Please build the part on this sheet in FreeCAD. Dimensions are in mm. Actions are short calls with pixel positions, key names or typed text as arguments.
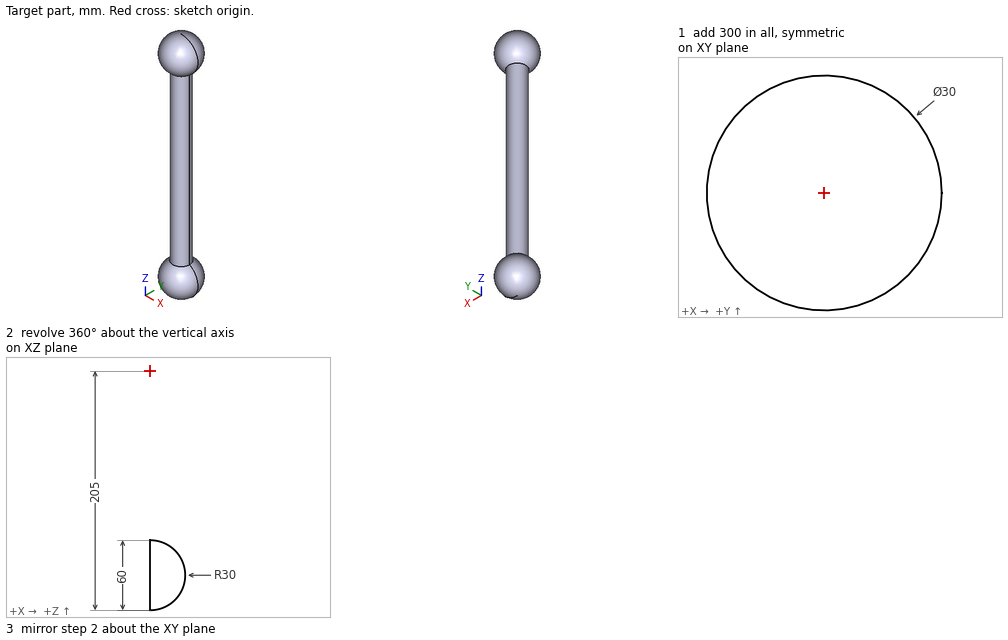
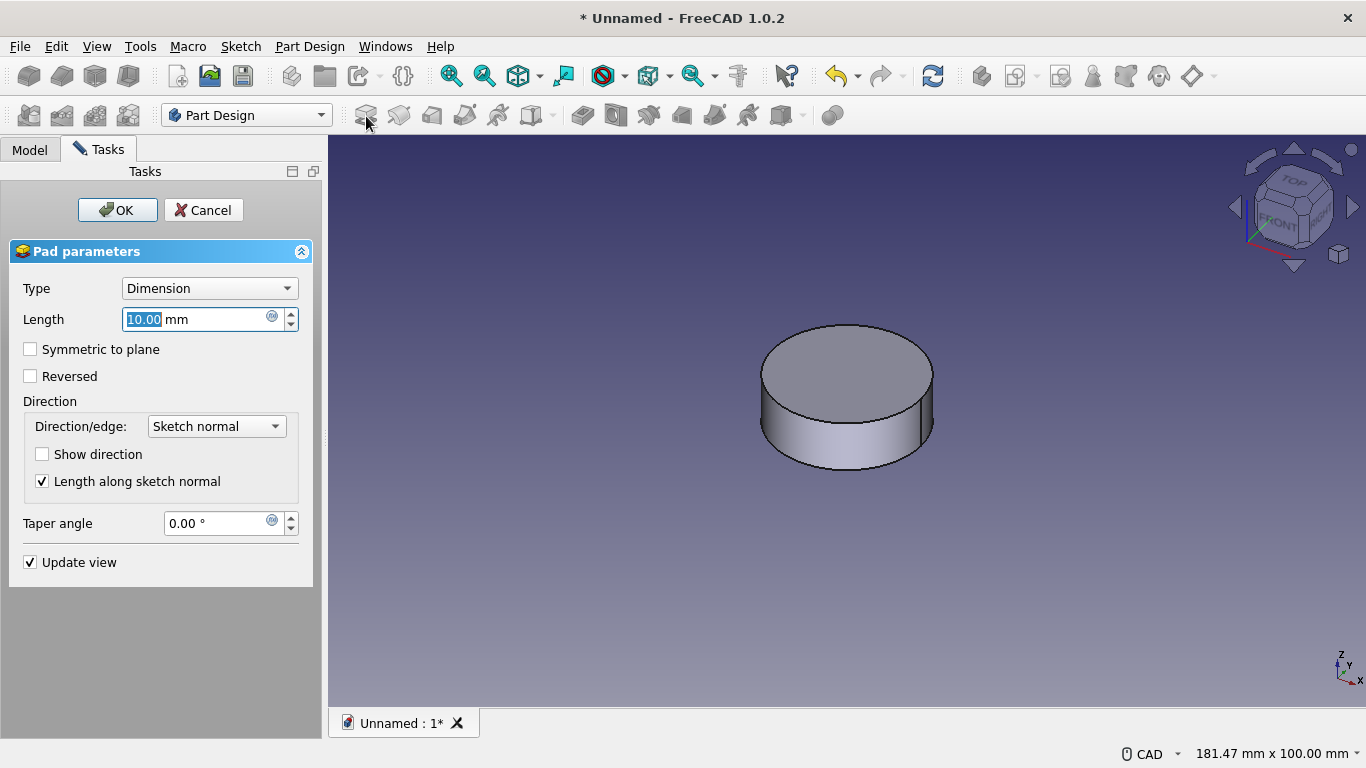
text(300)
key(Tab)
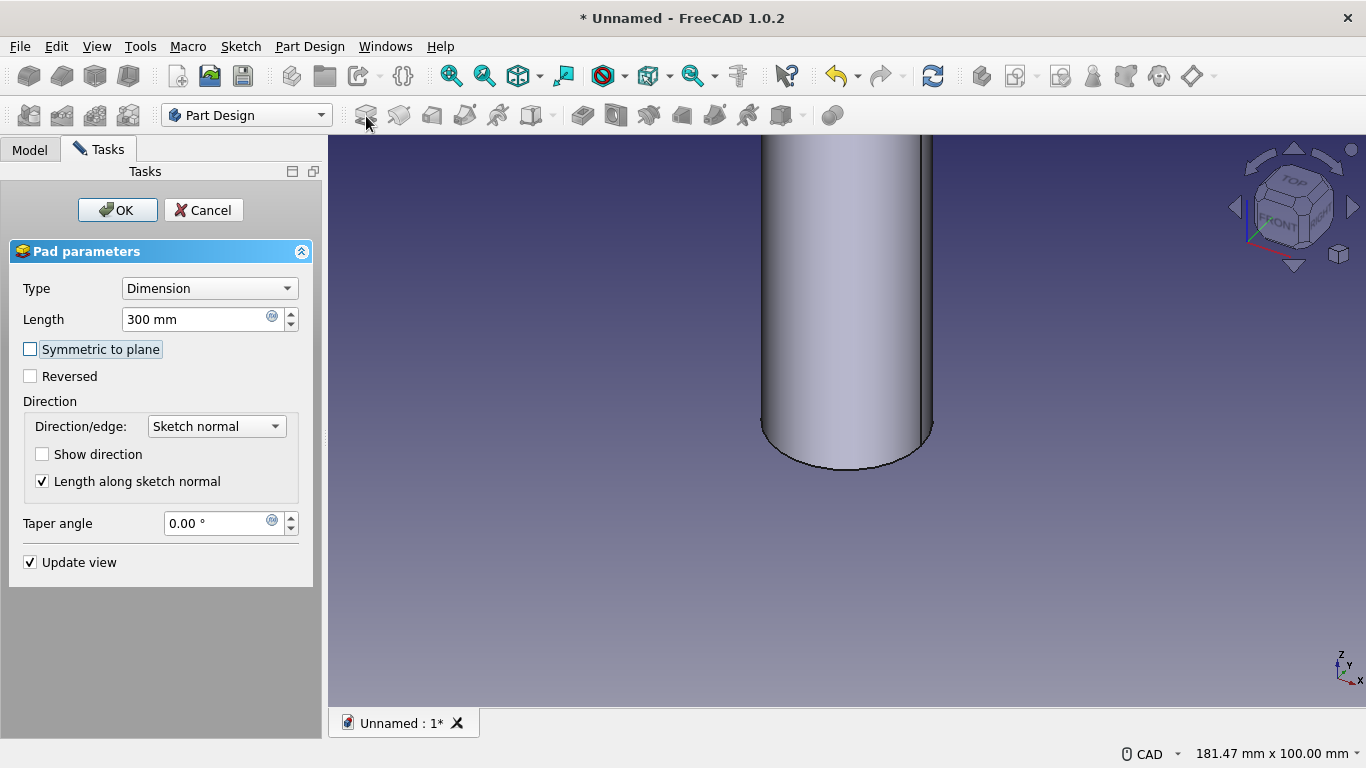
click(31, 349)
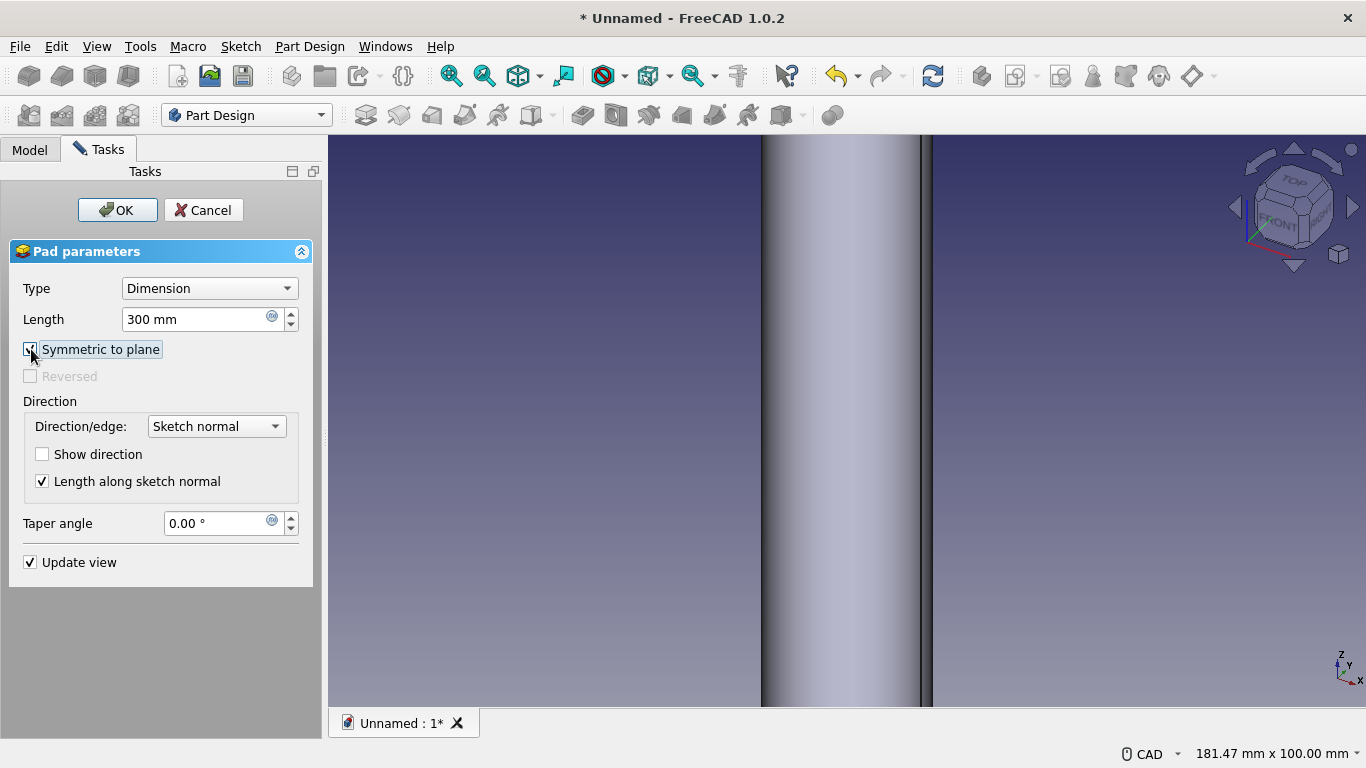
click(118, 210)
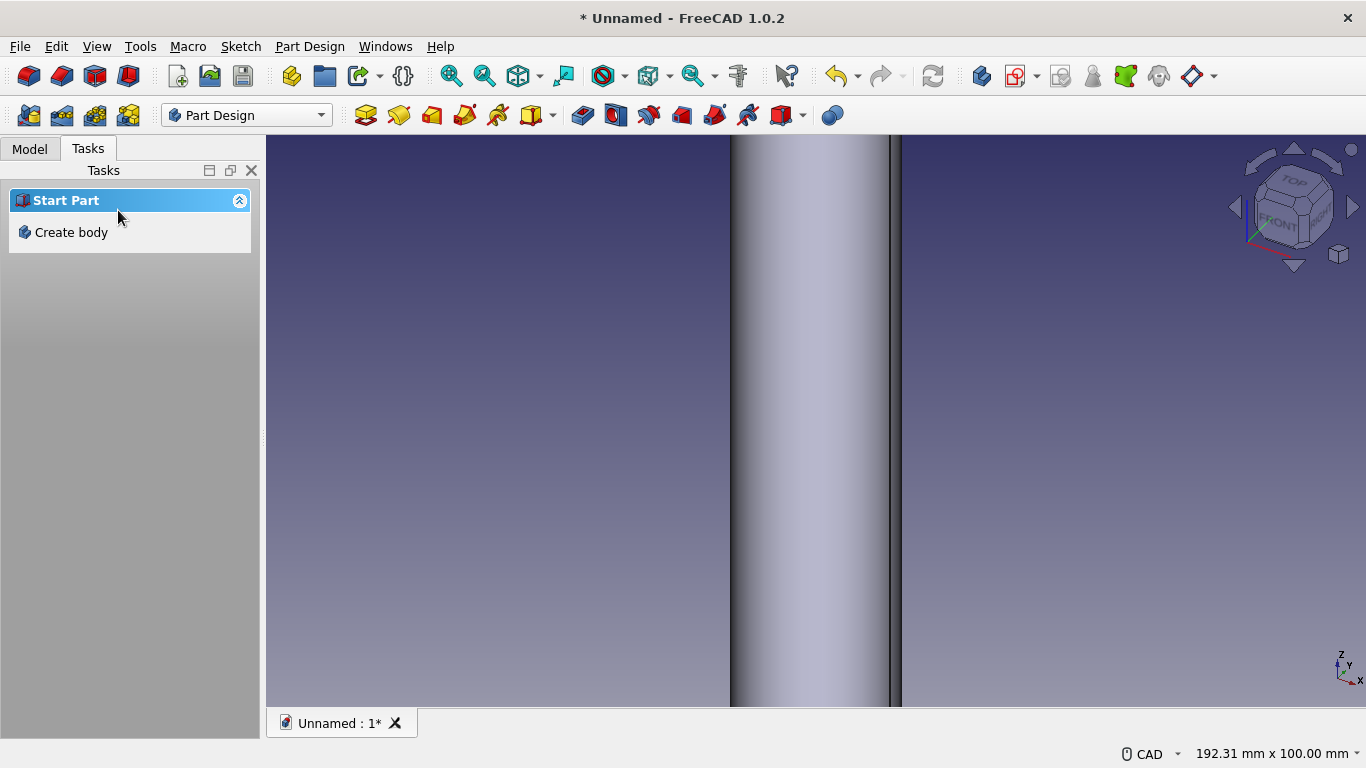
click(452, 76)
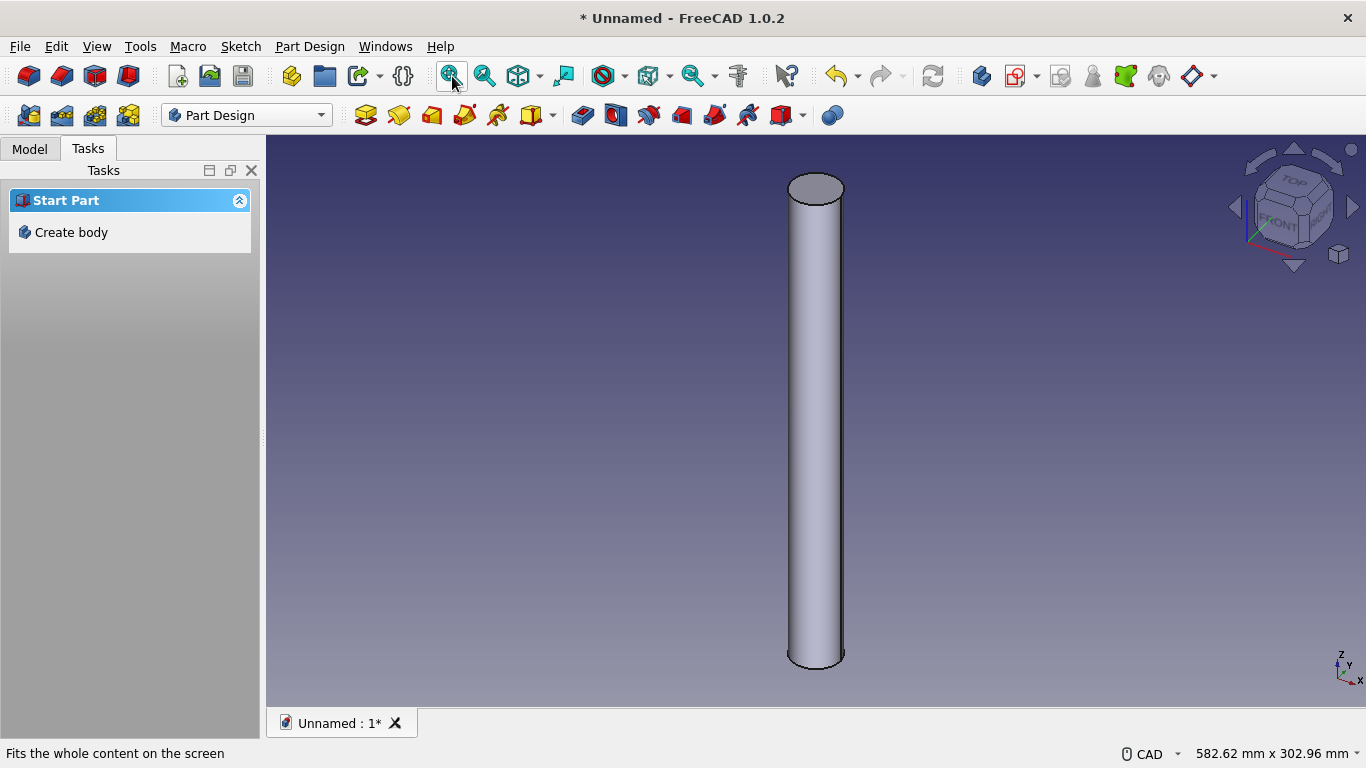
click(1014, 76)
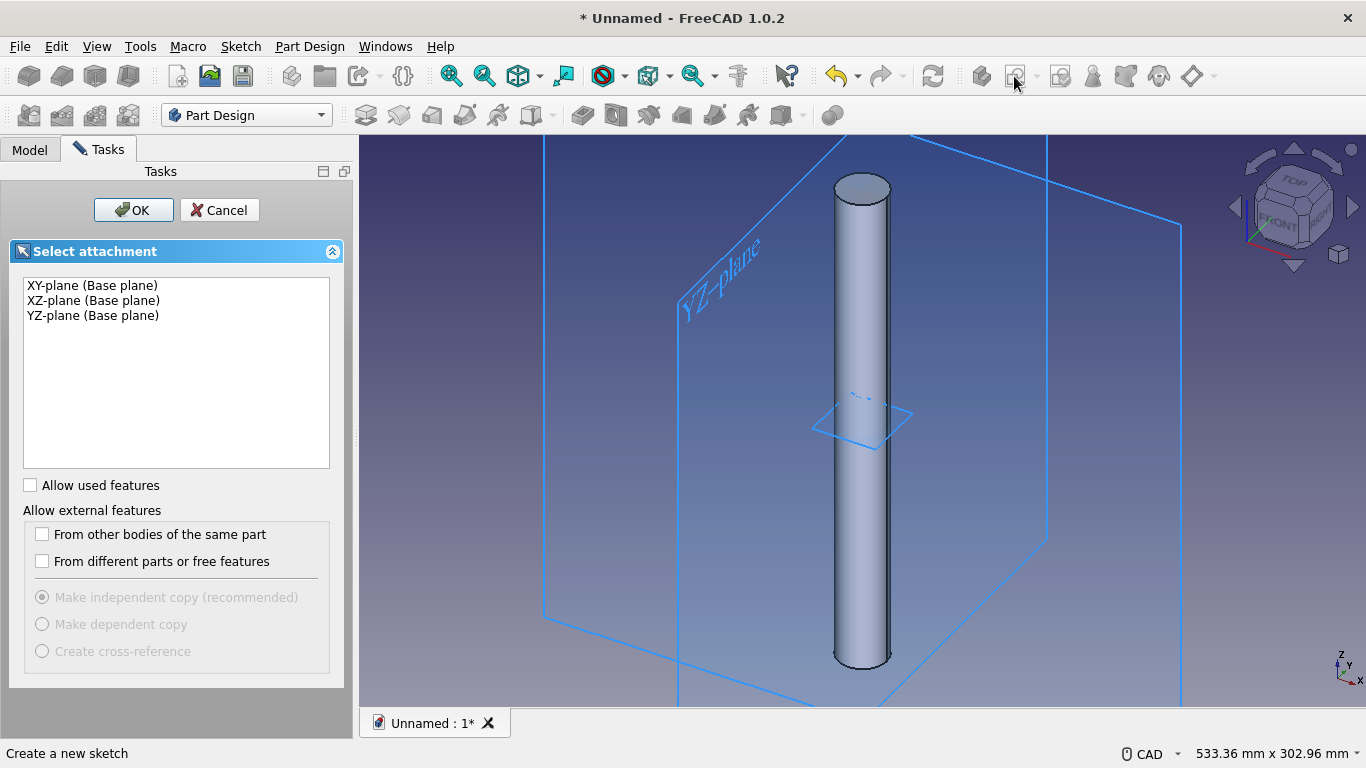
click(84, 300)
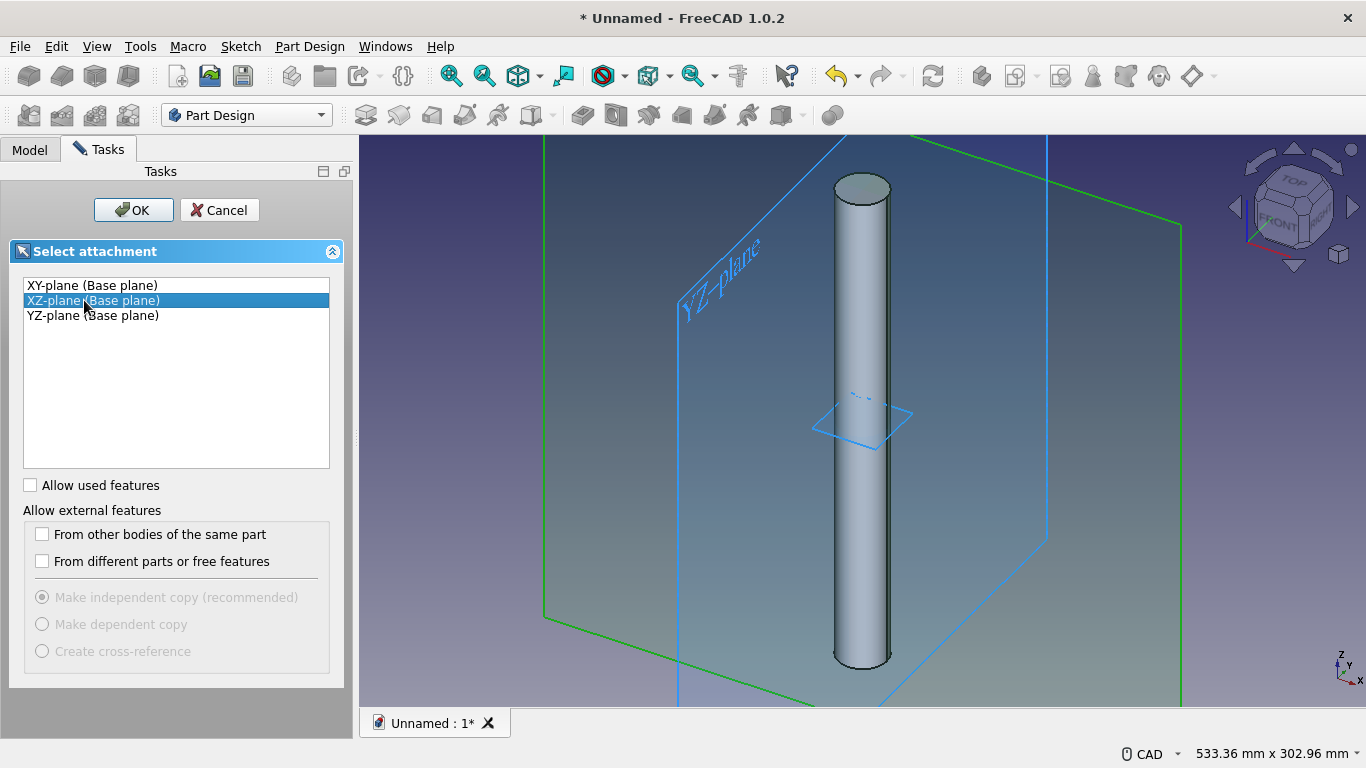
click(134, 210)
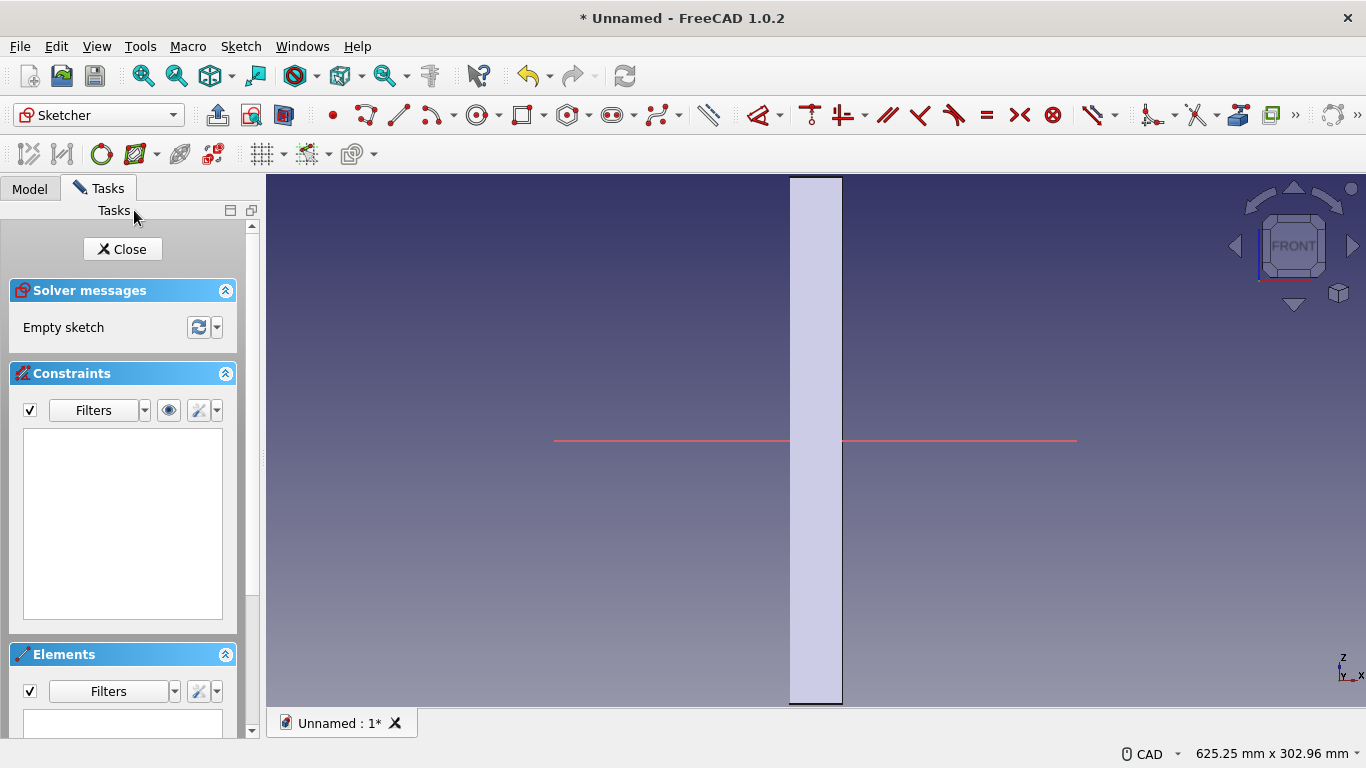
click(284, 116)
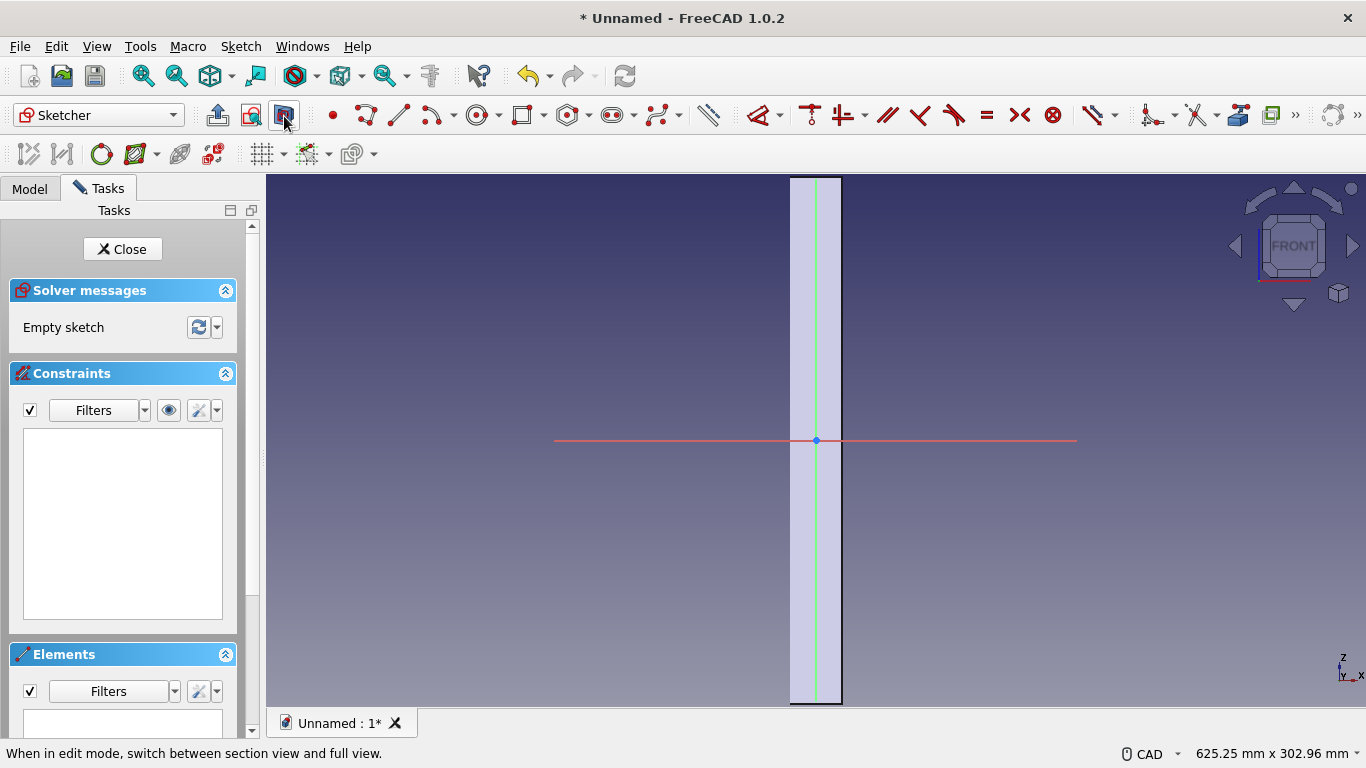
scroll(748, 440, down, 5)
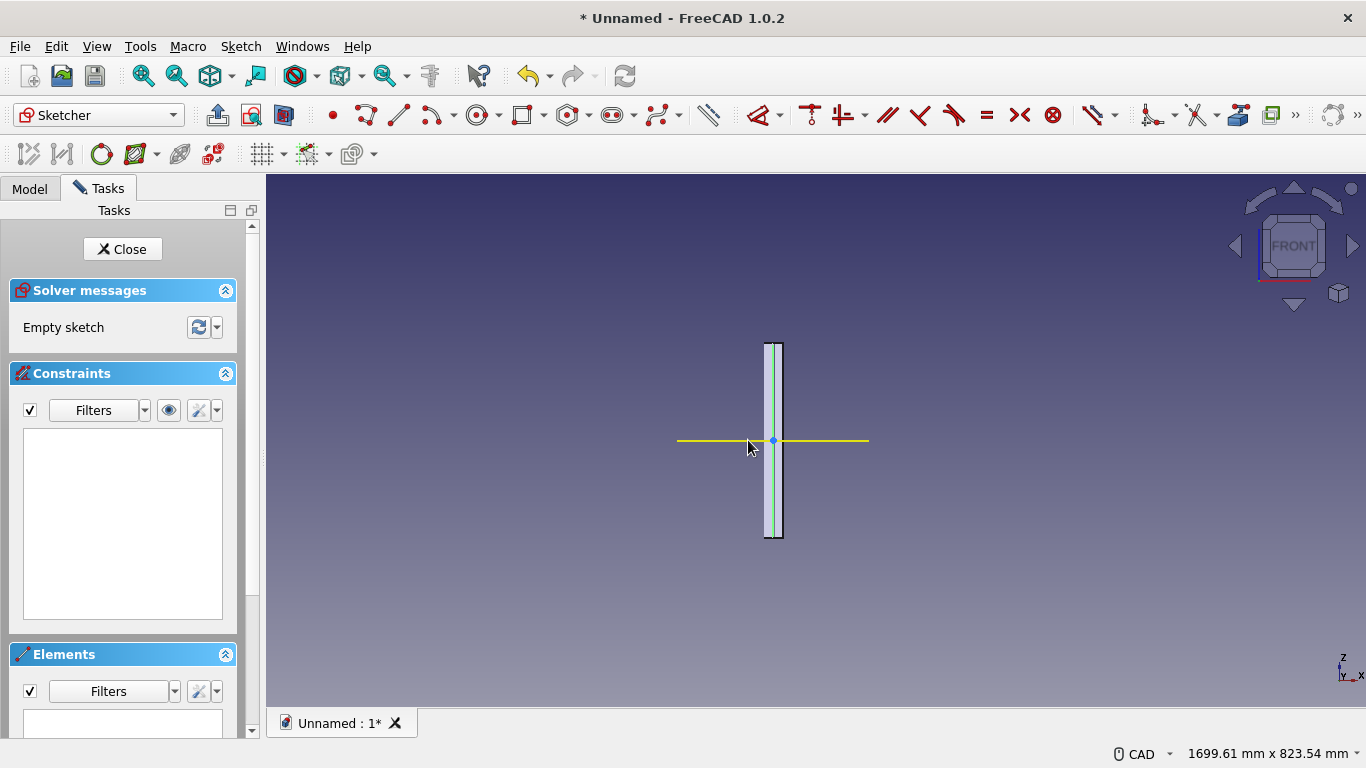
scroll(787, 568, up, 11)